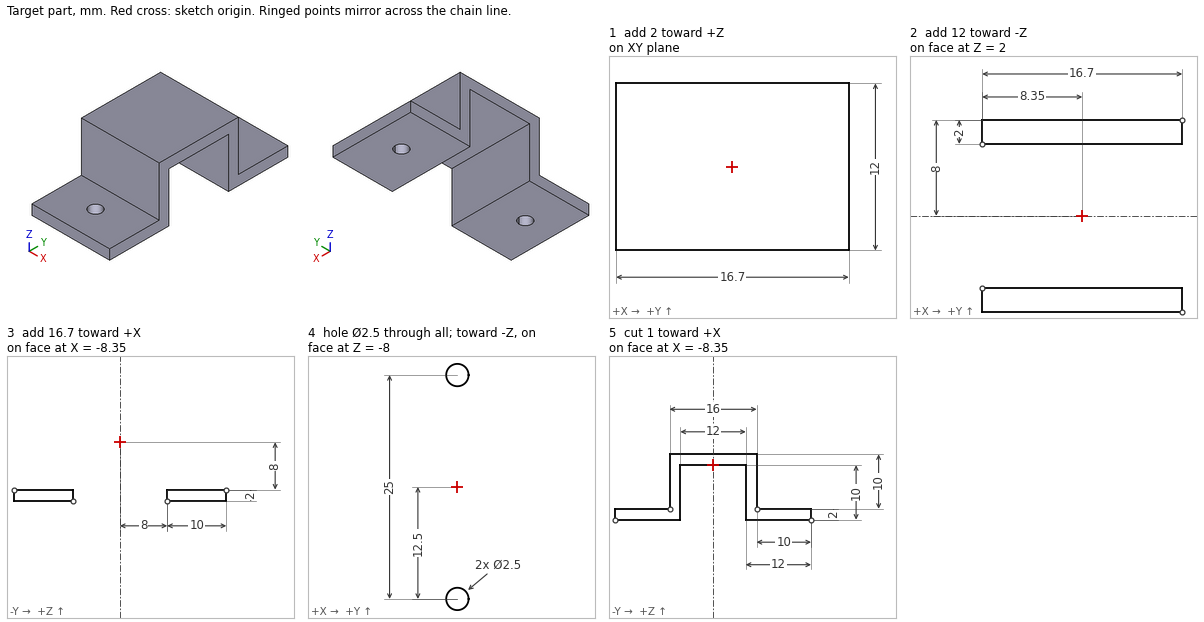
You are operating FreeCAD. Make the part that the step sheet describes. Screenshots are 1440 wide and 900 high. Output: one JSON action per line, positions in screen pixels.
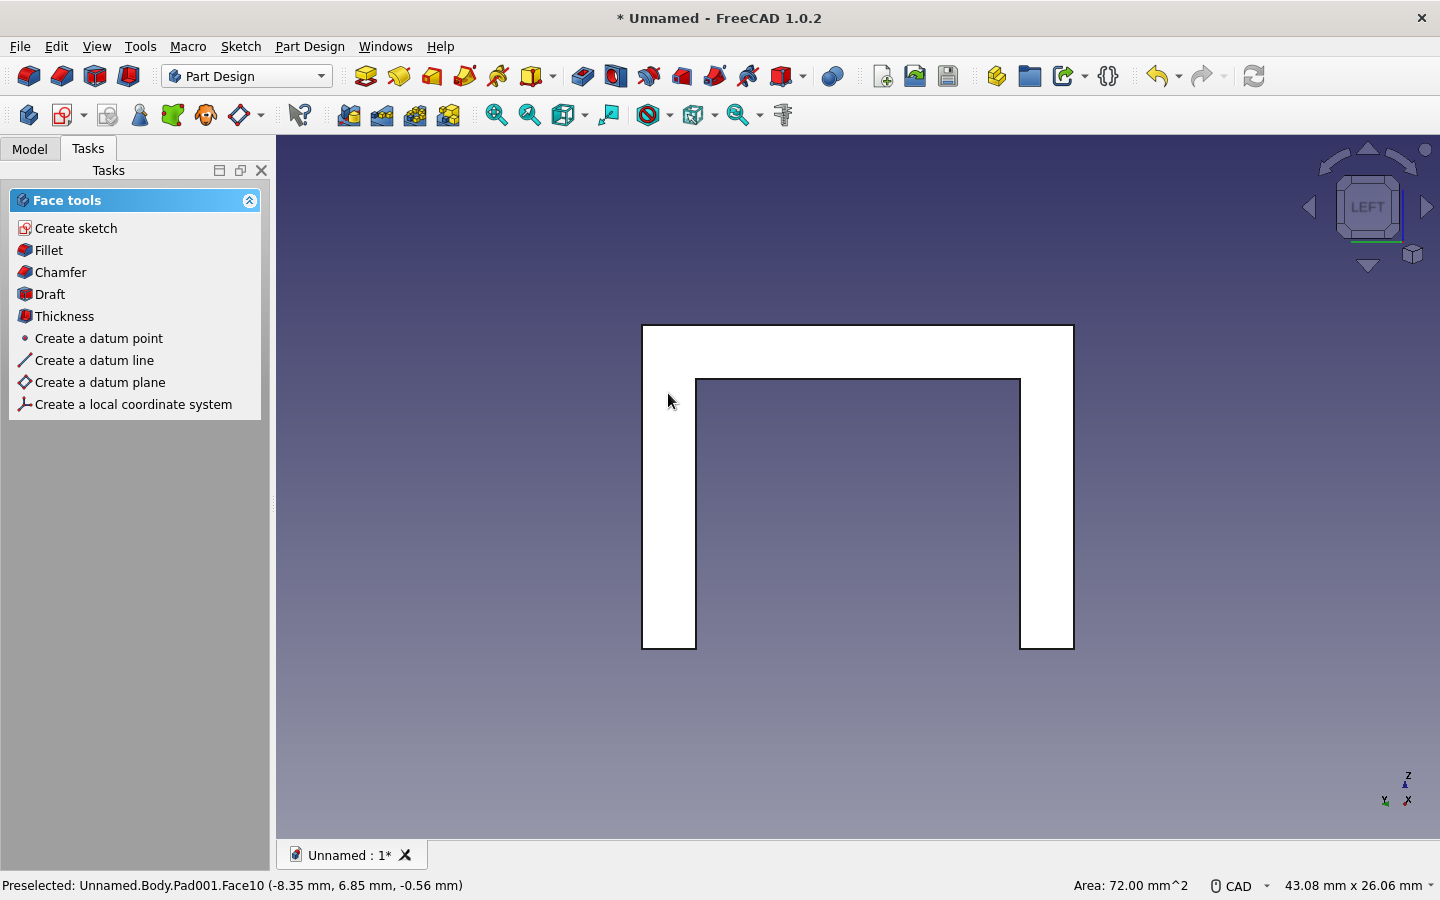
{"action": "left_click", "coordinate": [62, 116]}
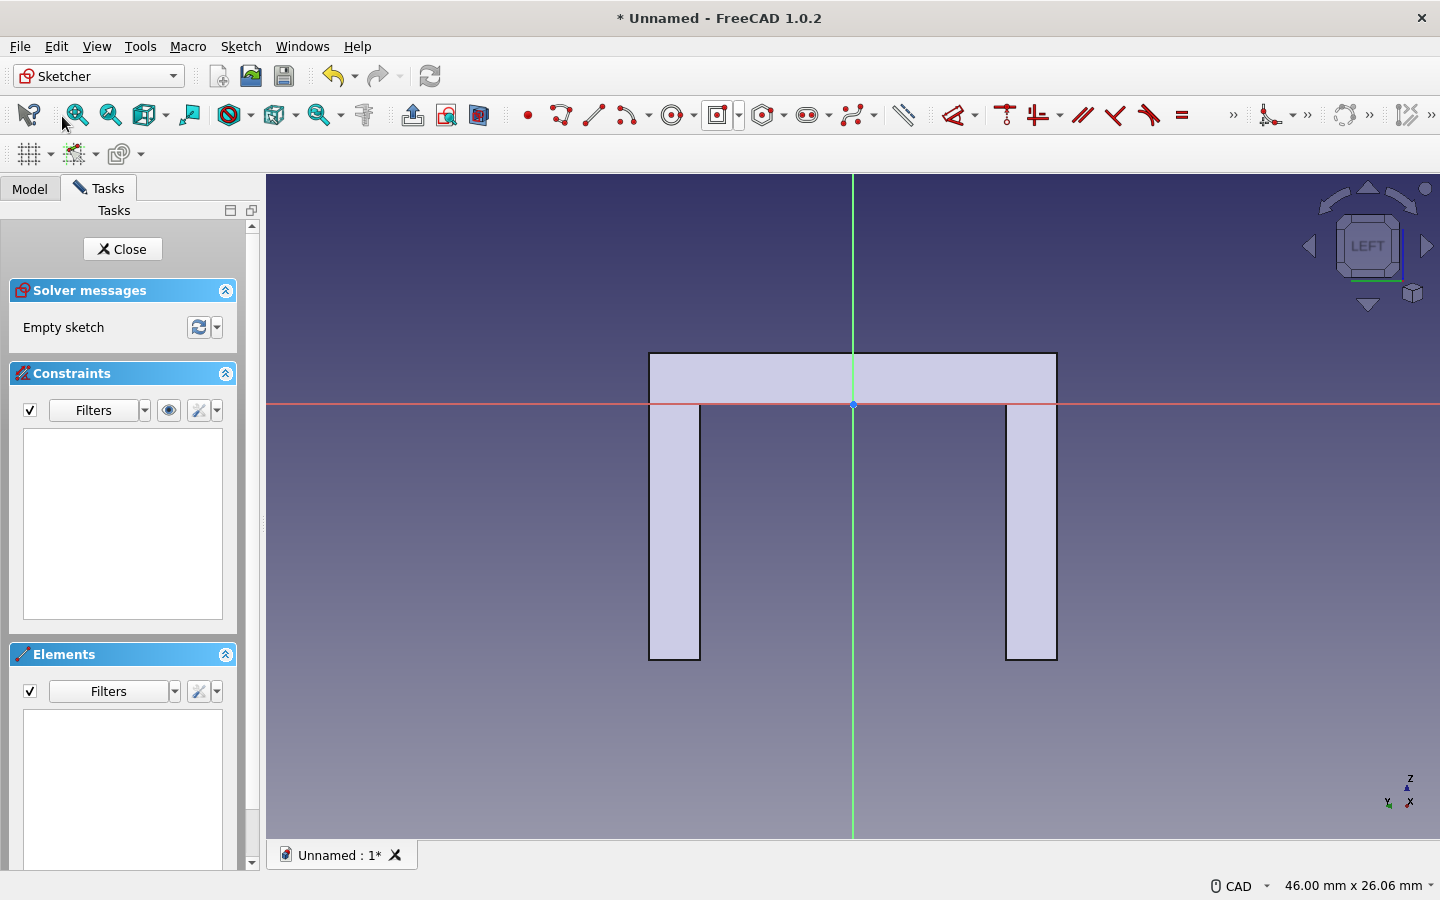
{"action": "scroll", "coordinate": [475, 391], "scroll_direction": "down", "scroll_amount": 1}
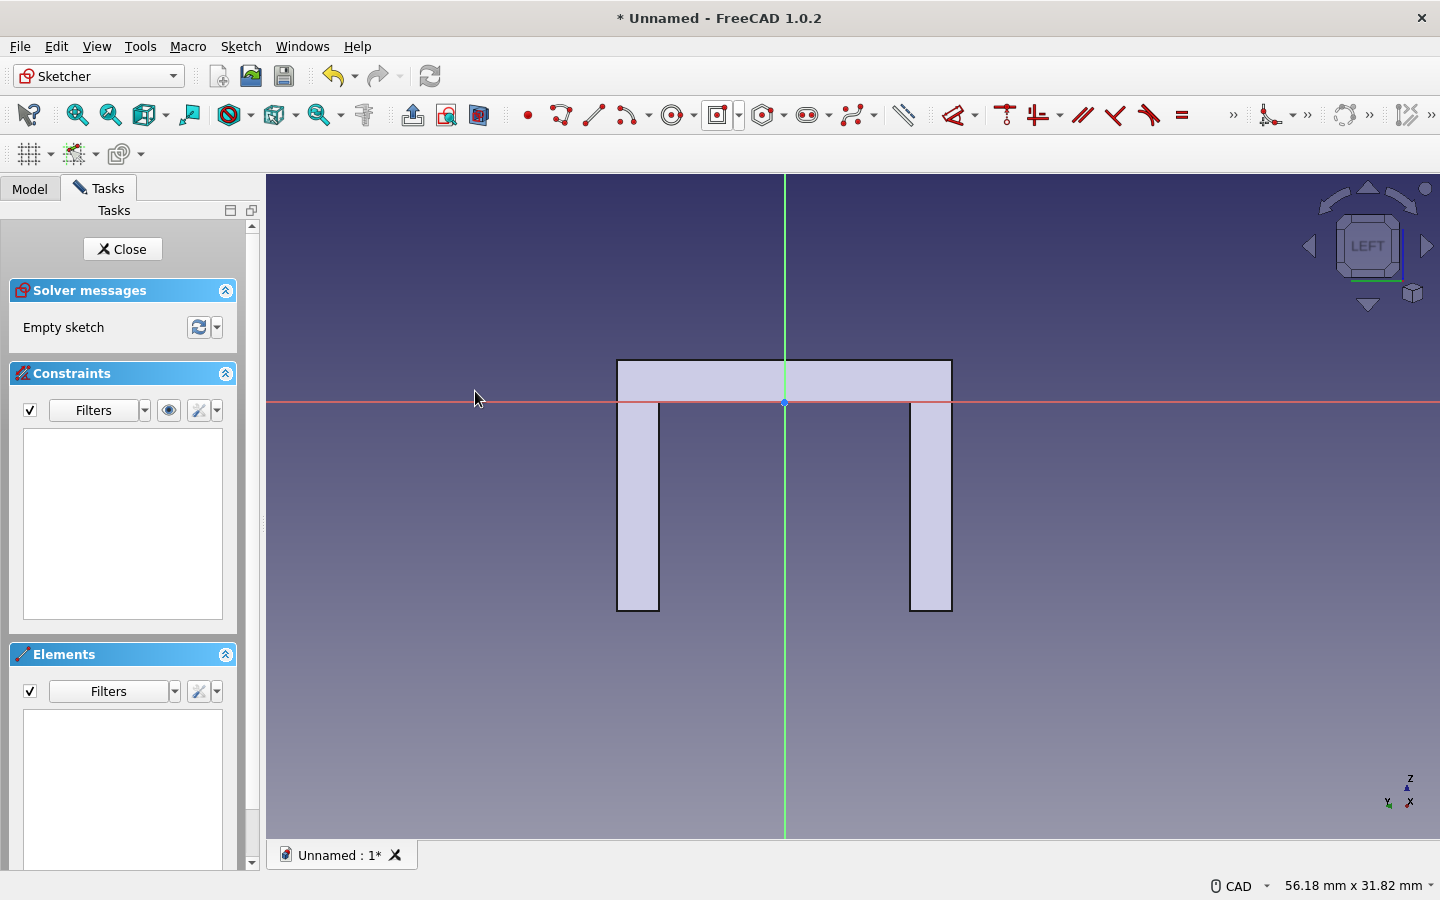
{"action": "left_click", "coordinate": [738, 116]}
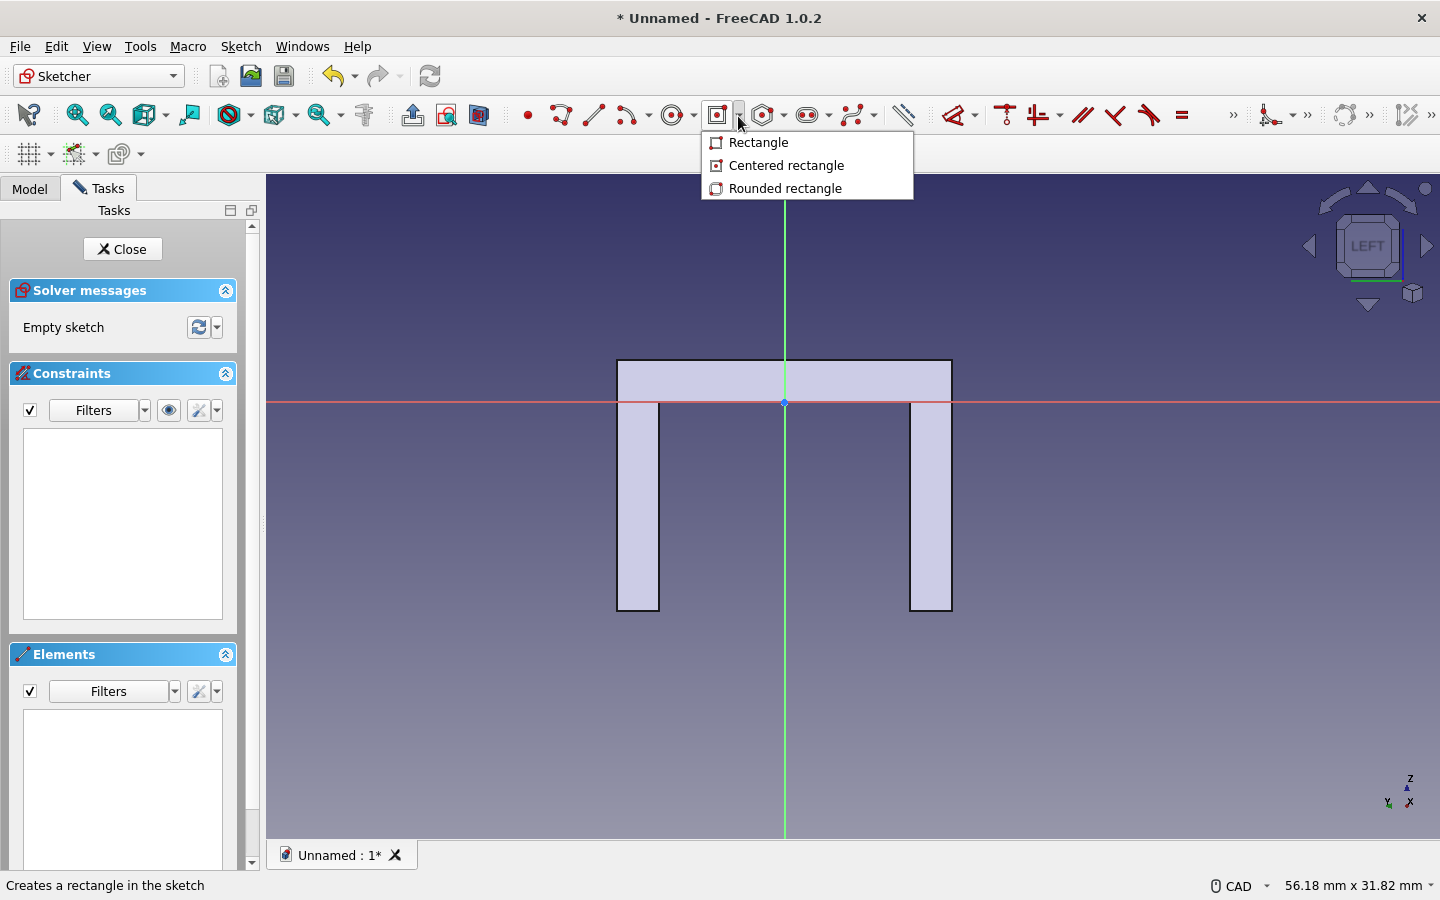
{"action": "left_click", "coordinate": [808, 142]}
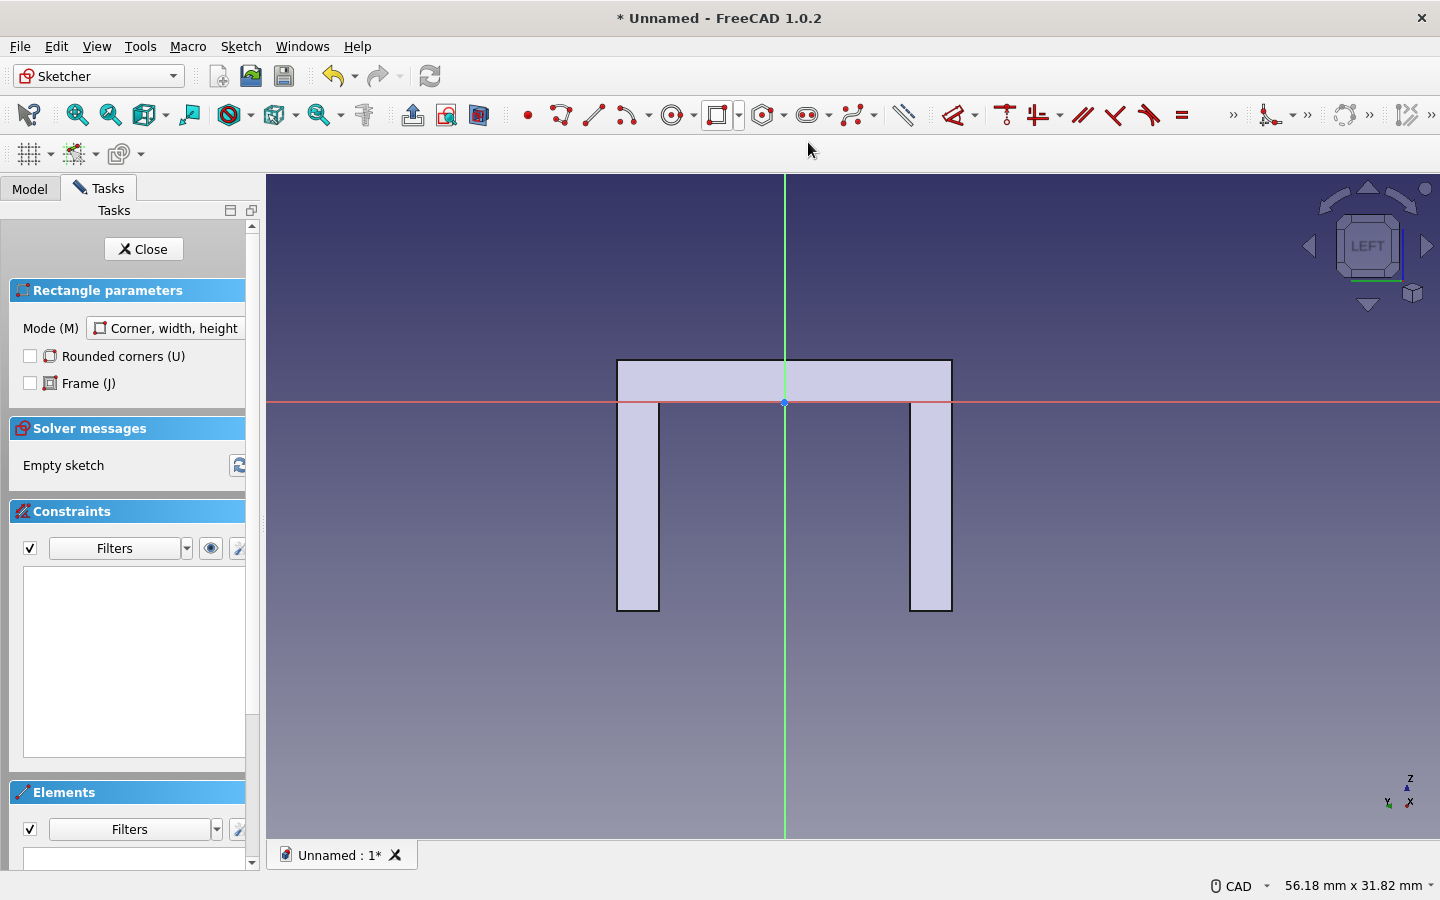
{"action": "left_click", "coordinate": [952, 569]}
{"action": "left_click", "coordinate": [1161, 611]}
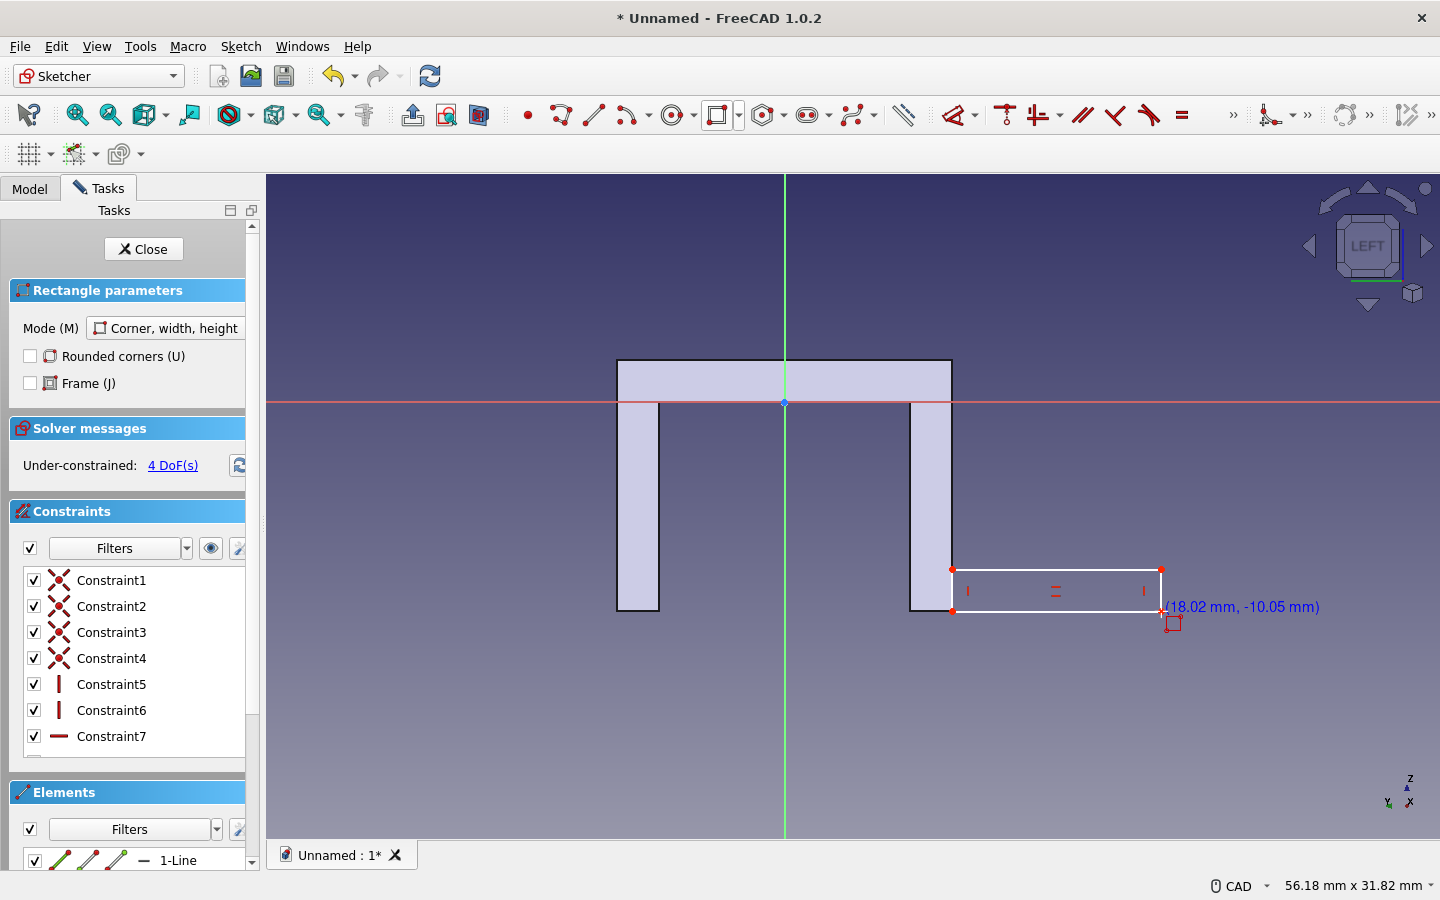
{"action": "left_click", "coordinate": [408, 569]}
{"action": "left_click", "coordinate": [617, 611]}
{"action": "key", "text": "Escape"}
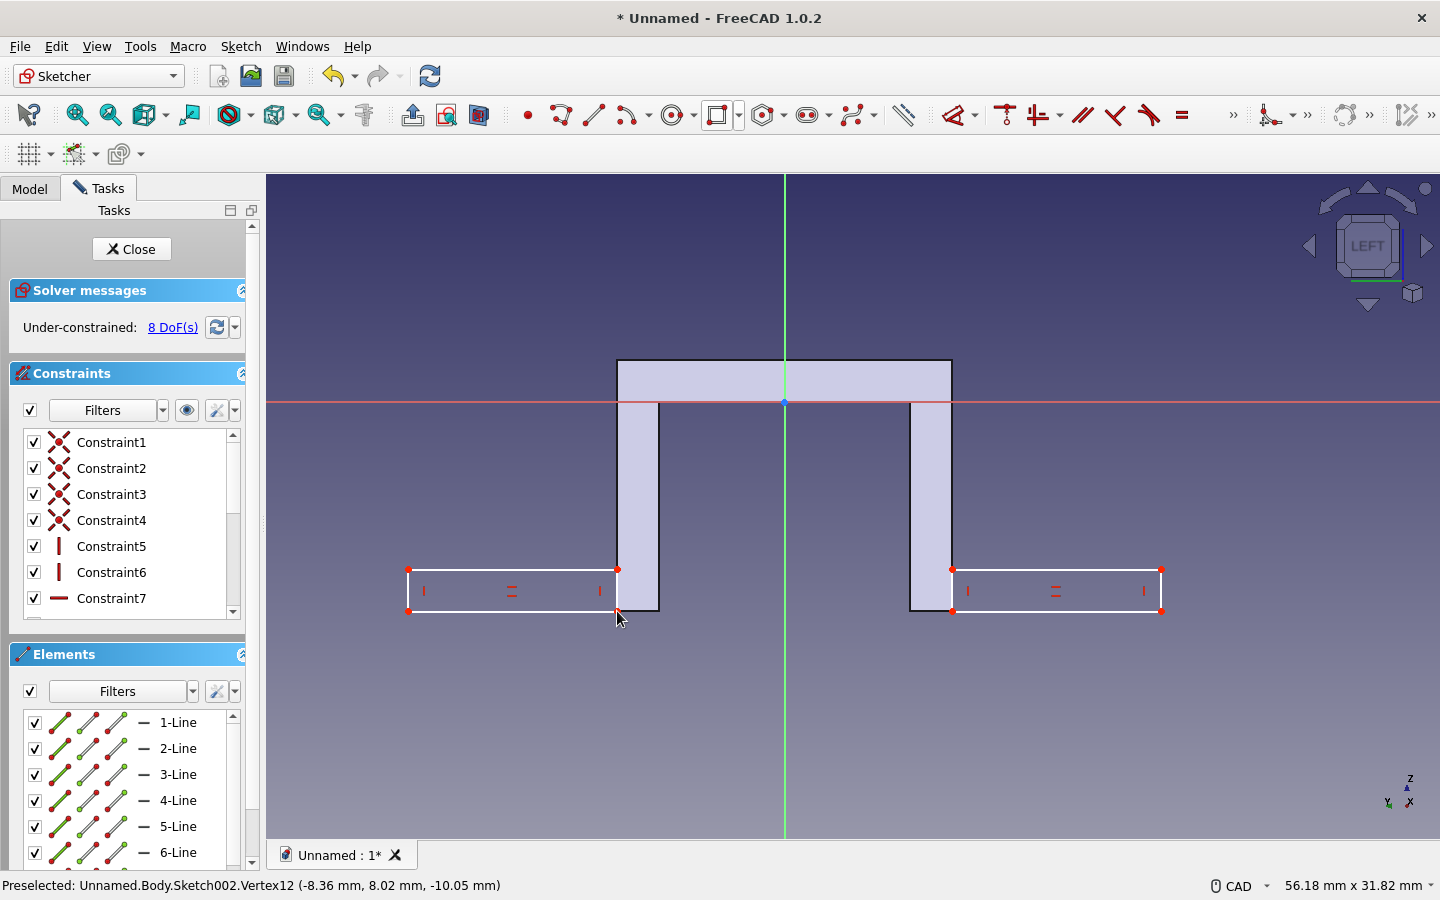
{"action": "left_click", "coordinate": [1161, 570]}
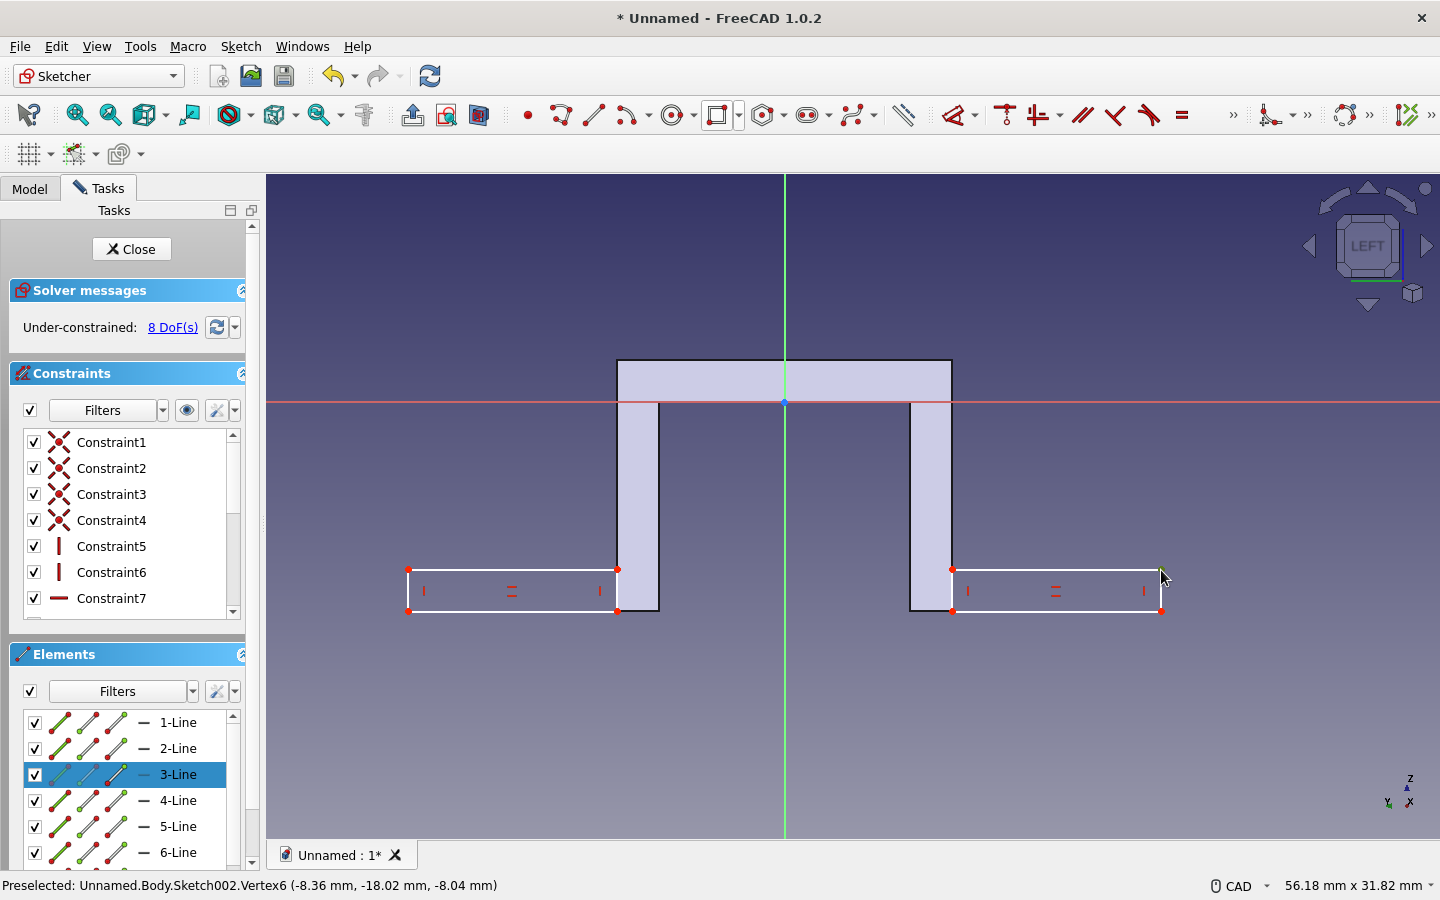
{"action": "left_click", "coordinate": [408, 570]}